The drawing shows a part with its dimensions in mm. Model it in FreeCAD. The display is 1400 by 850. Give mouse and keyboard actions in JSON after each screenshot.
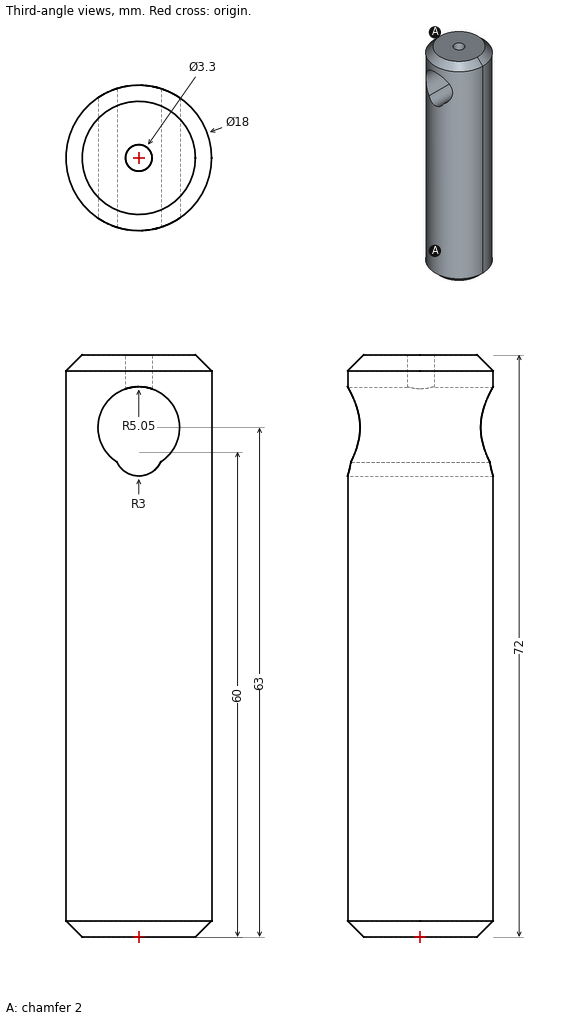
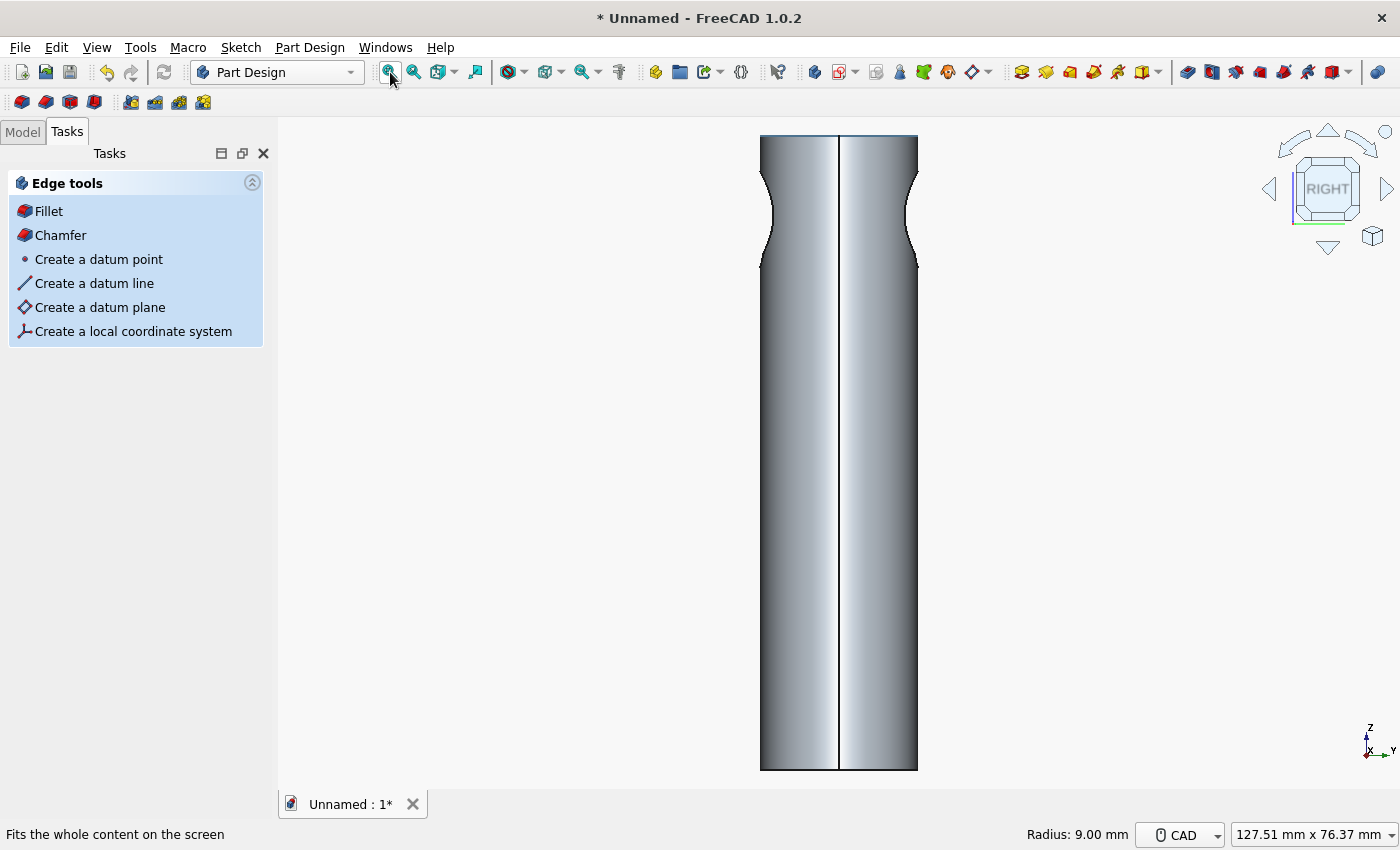
{"action": "key", "text": "5"}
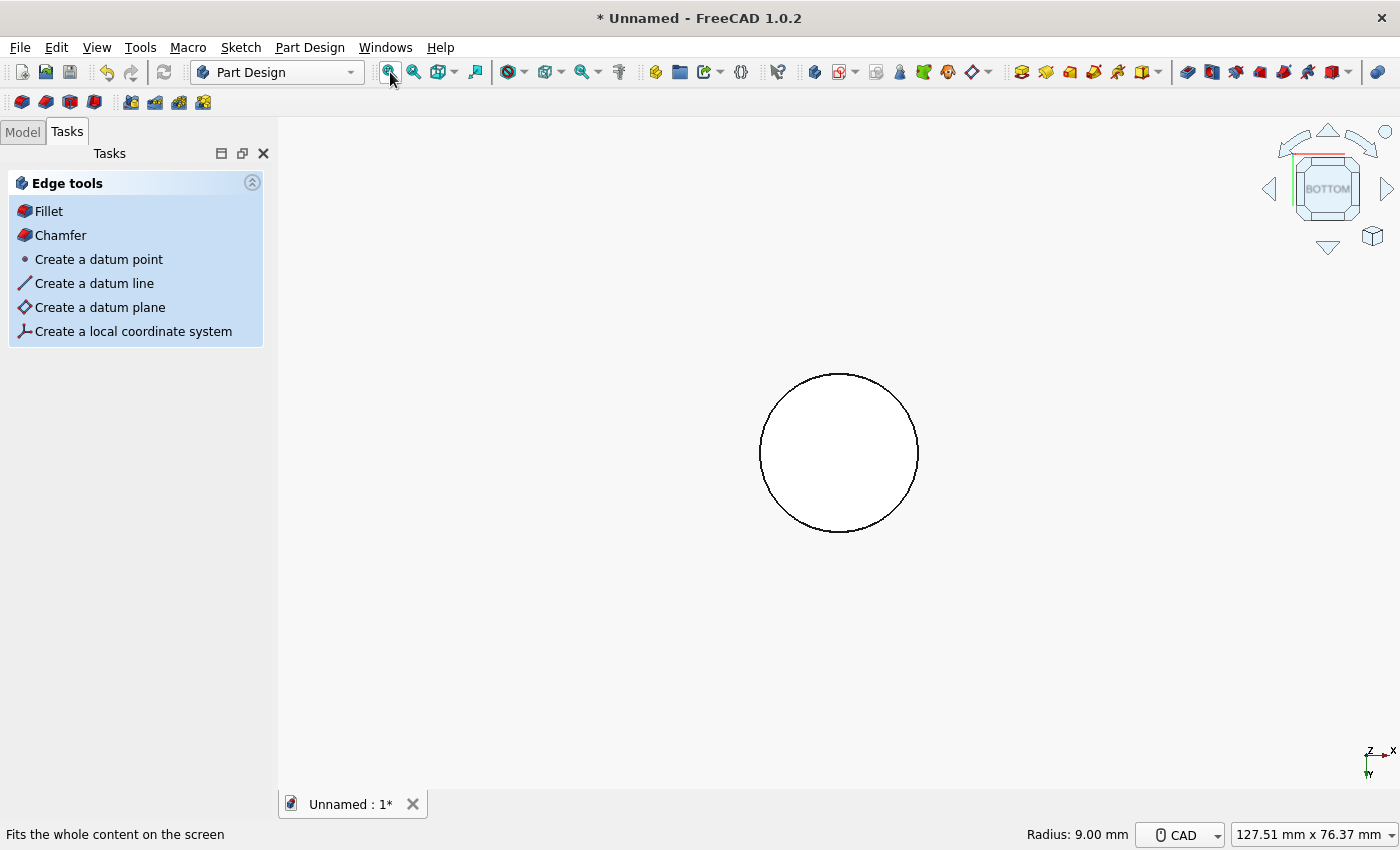
{"action": "left_click", "coordinate": [390, 72]}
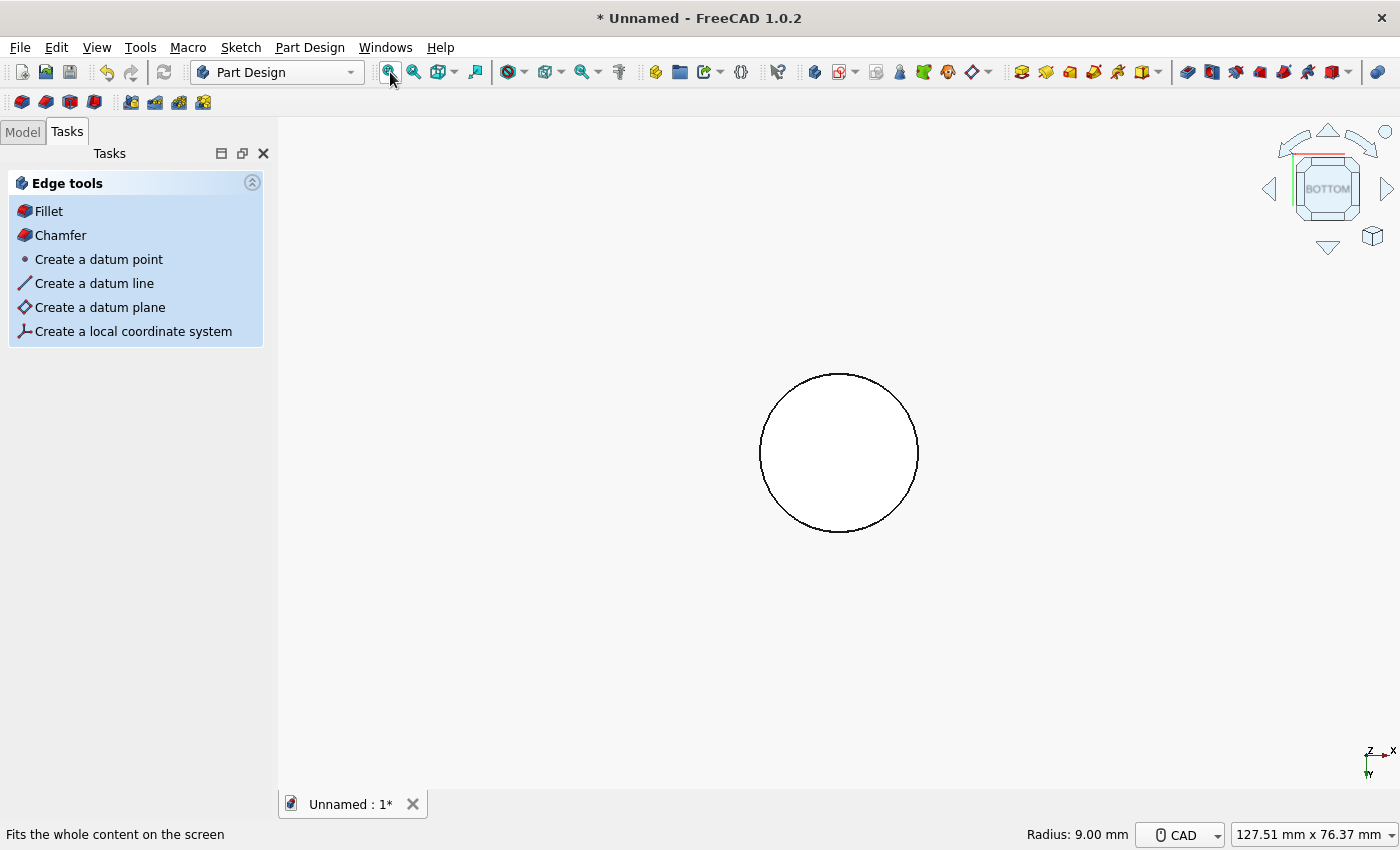
{"action": "left_click", "coordinate": [760, 452], "text": "ctrl"}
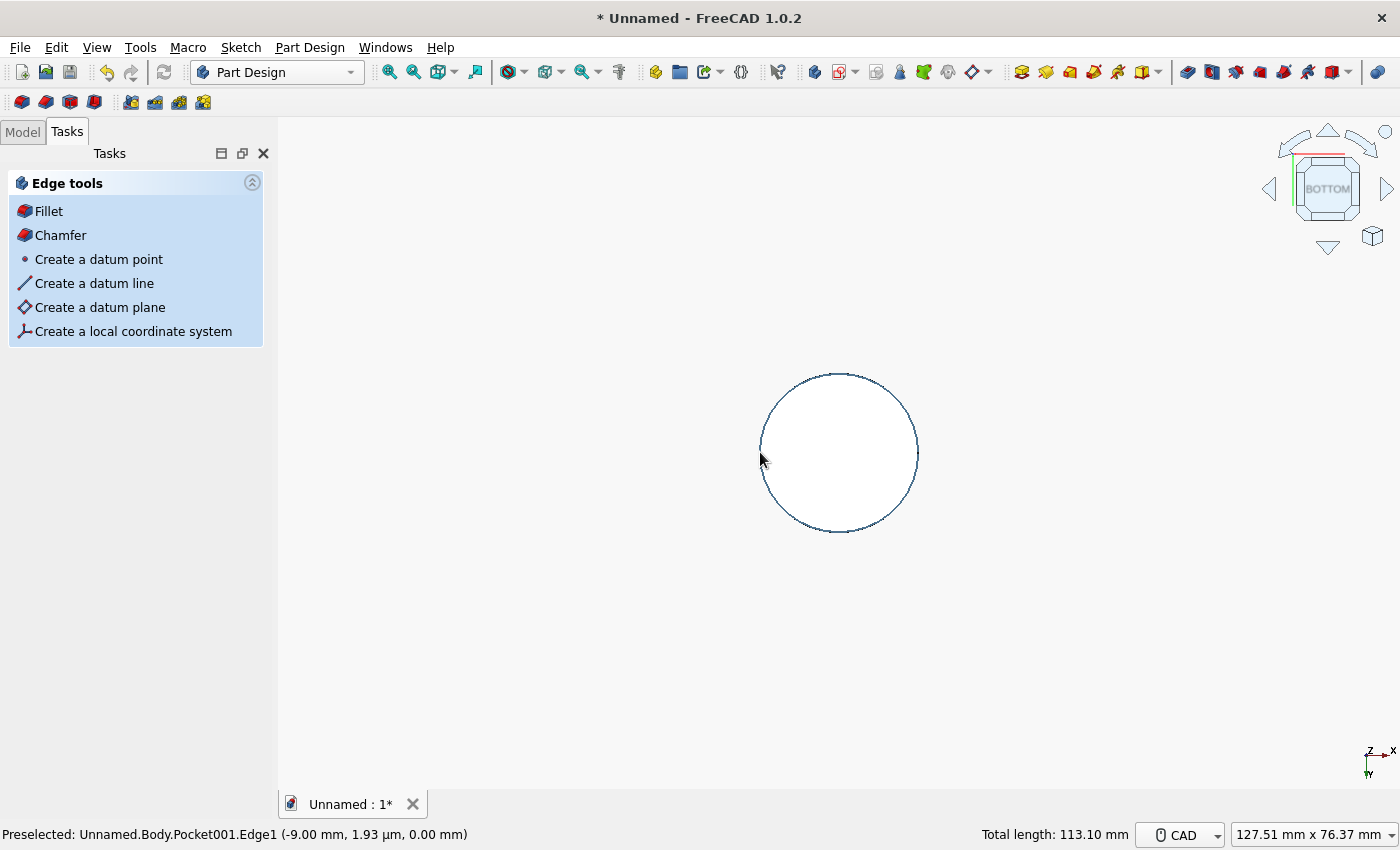
{"action": "left_click", "coordinate": [46, 102]}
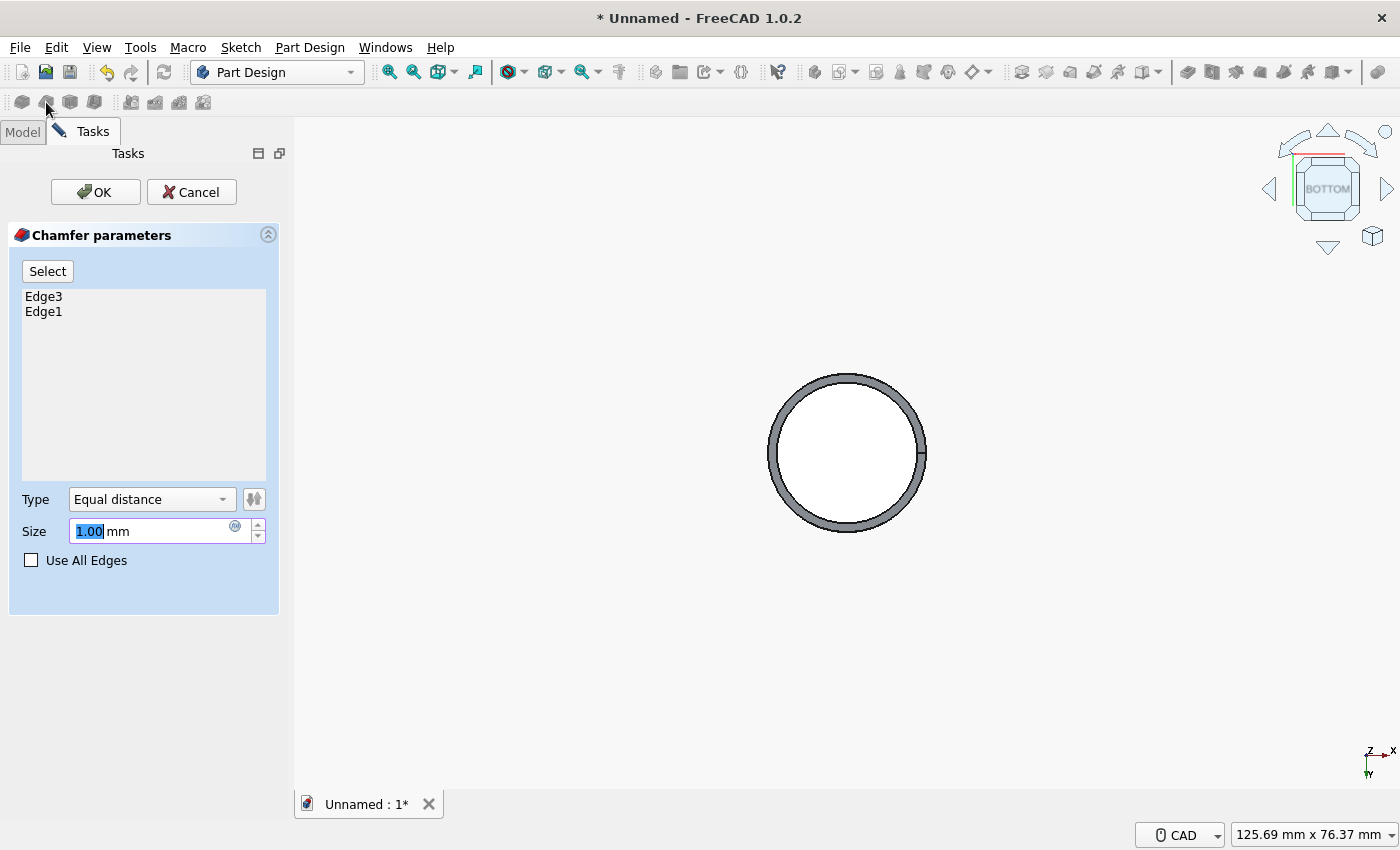
{"action": "type", "text": "2"}
{"action": "key", "text": "Tab"}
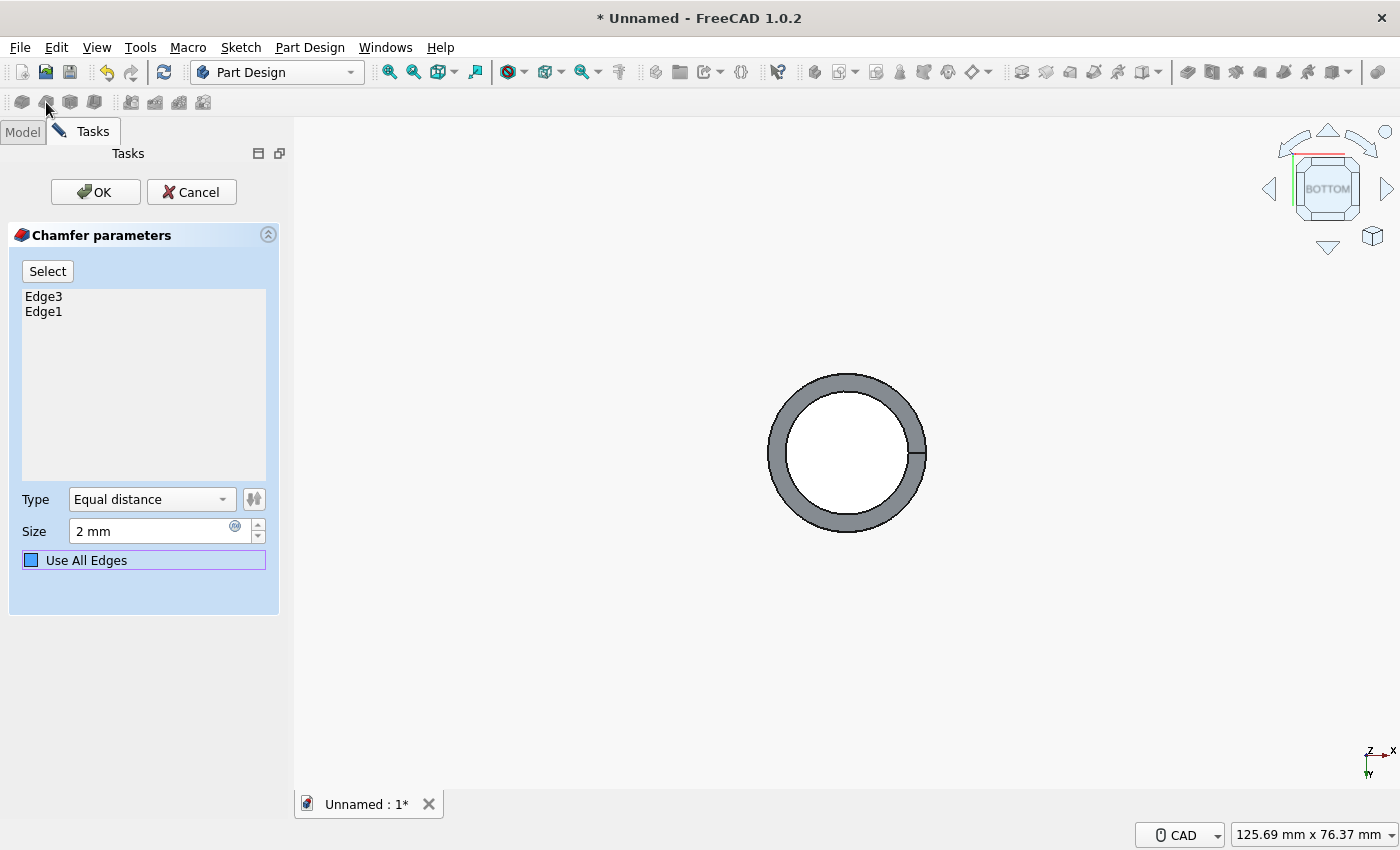
{"action": "left_click", "coordinate": [96, 192]}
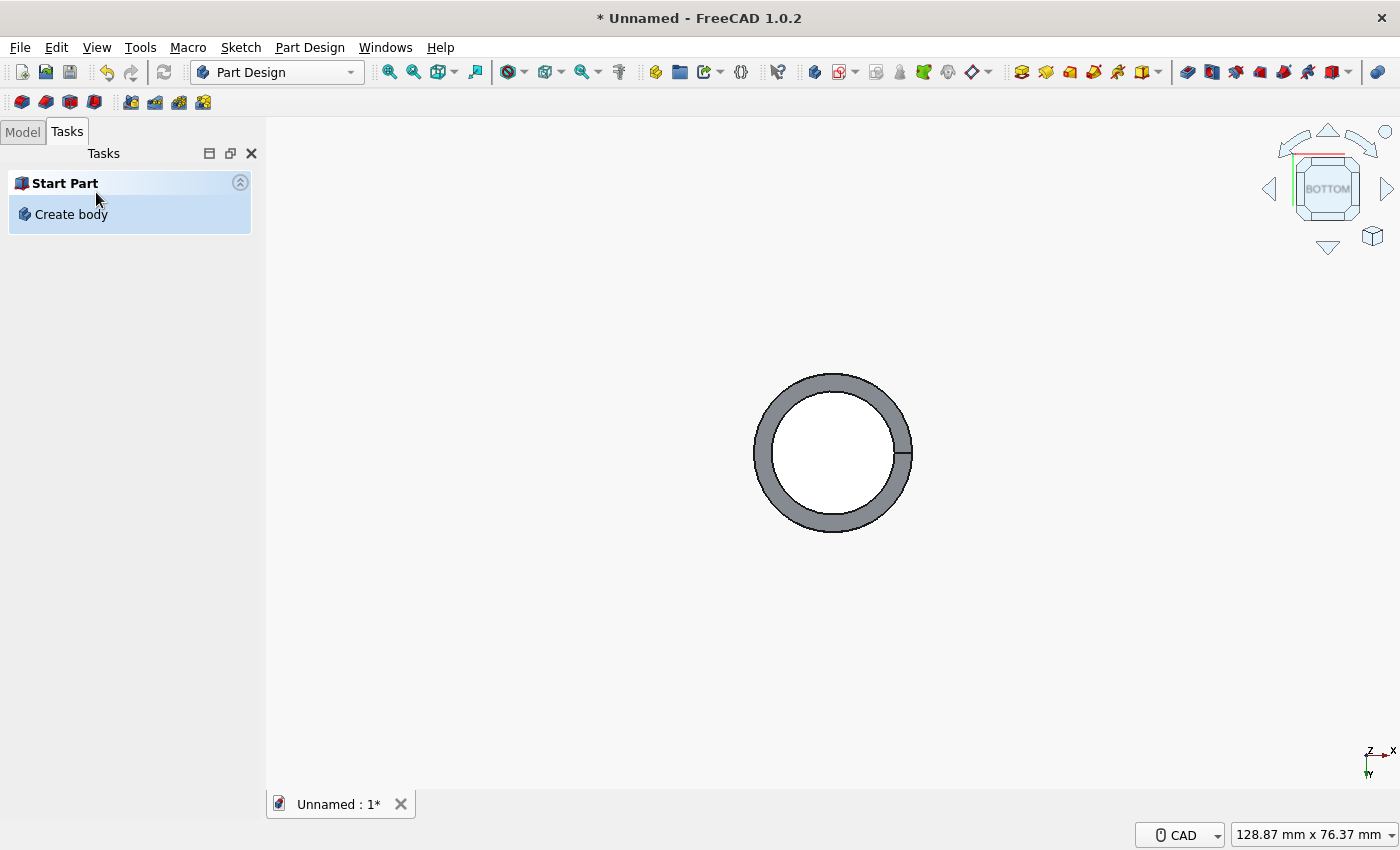
{"action": "key", "text": "0"}